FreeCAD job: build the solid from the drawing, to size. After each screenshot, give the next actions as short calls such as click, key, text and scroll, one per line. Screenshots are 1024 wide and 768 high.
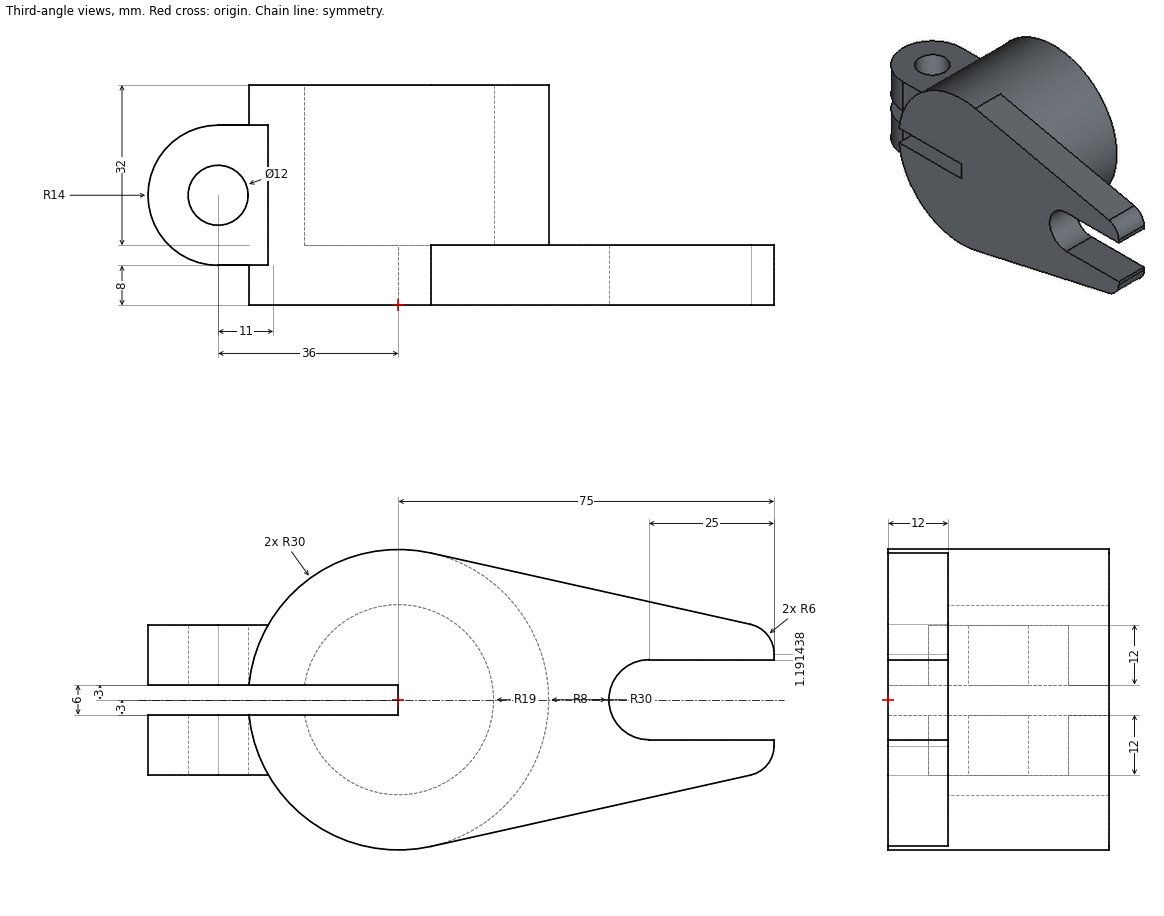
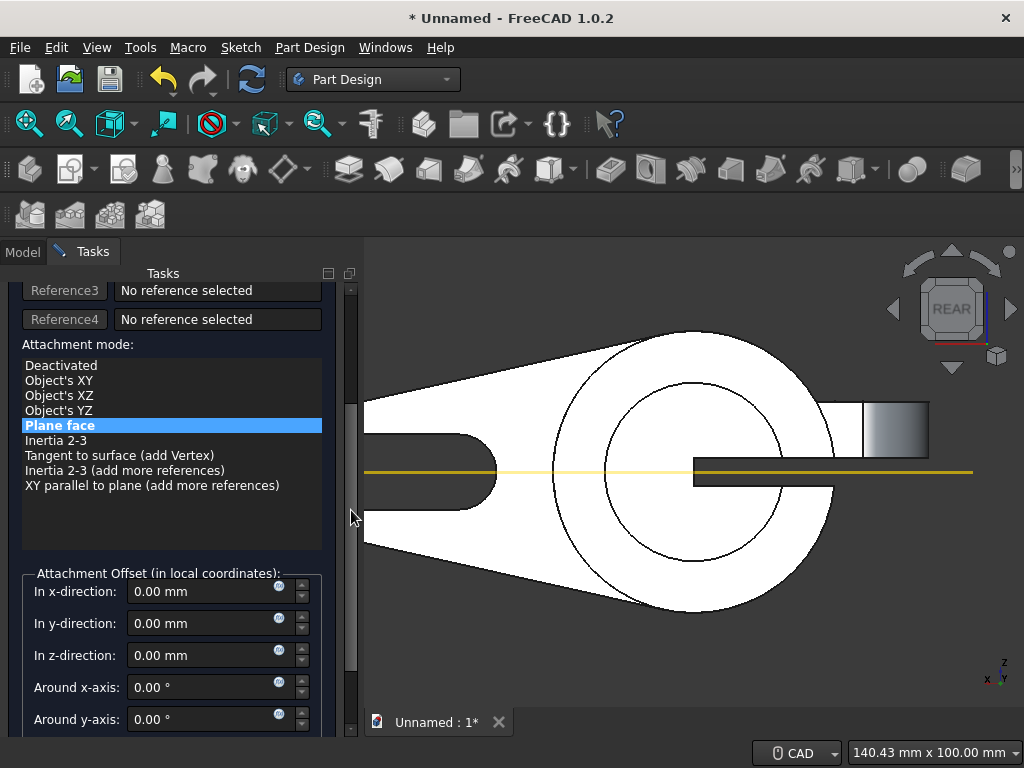
triple_click(210, 655)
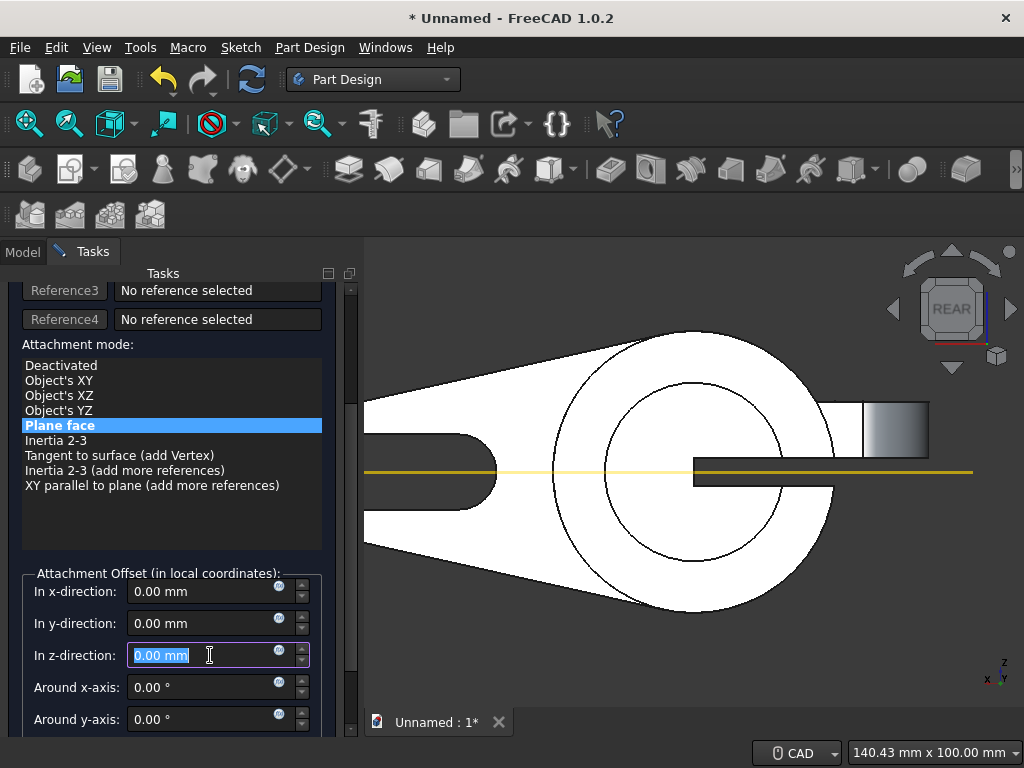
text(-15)
key(Tab)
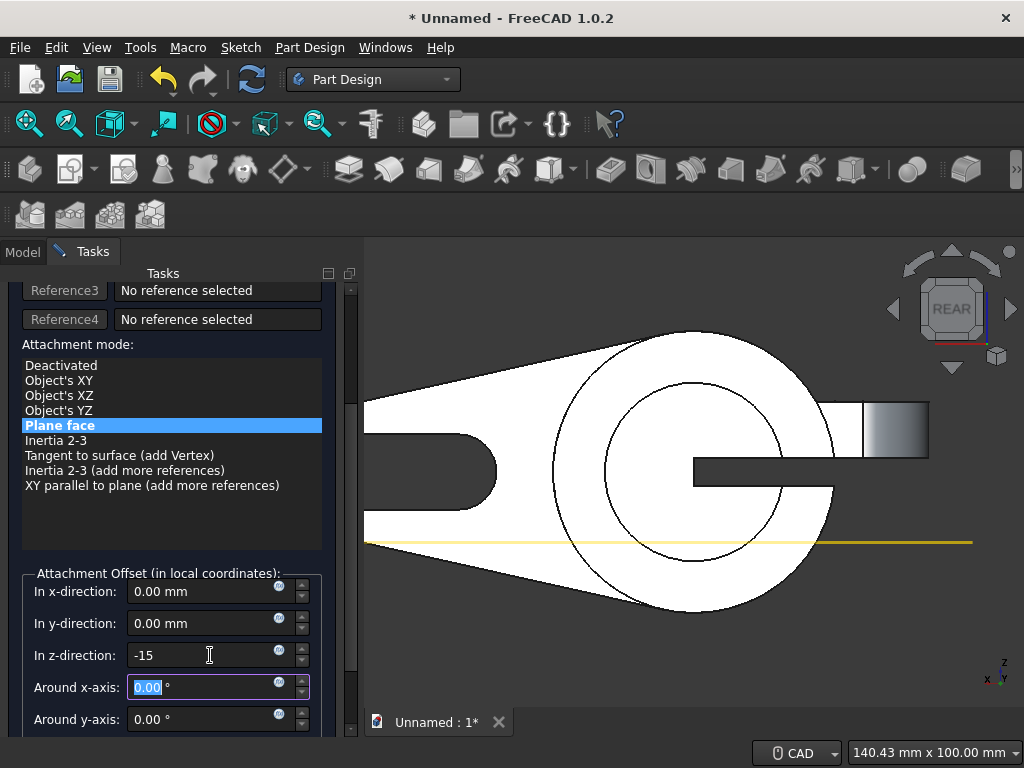
scroll(351, 510, up, 4)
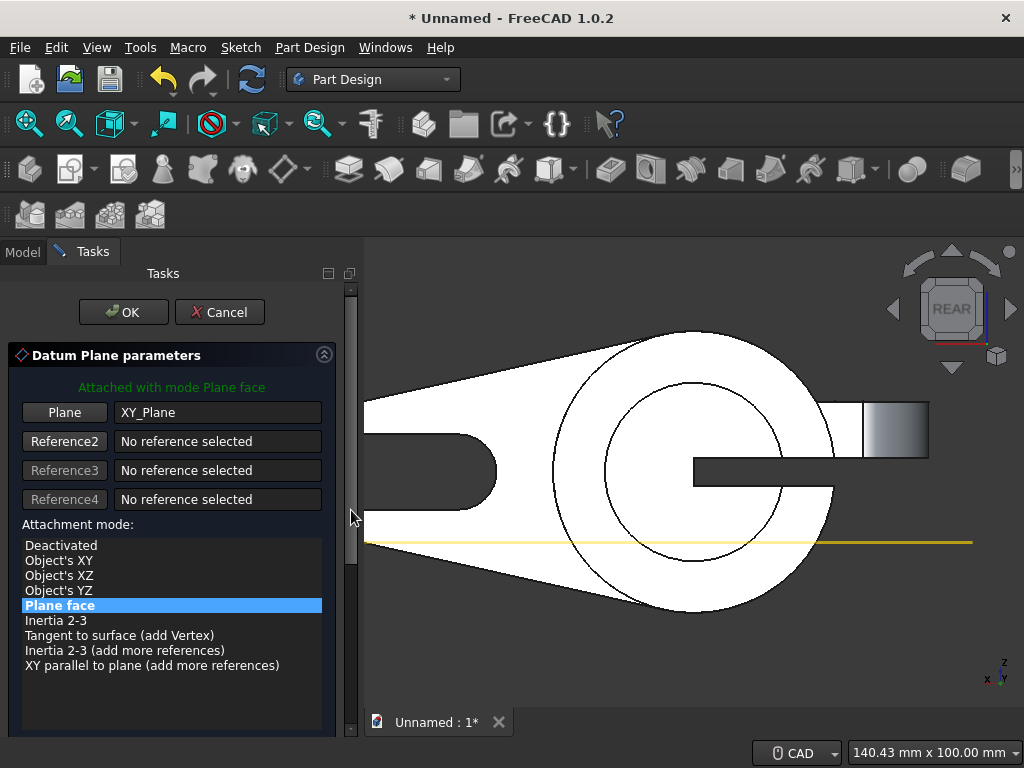
click(124, 312)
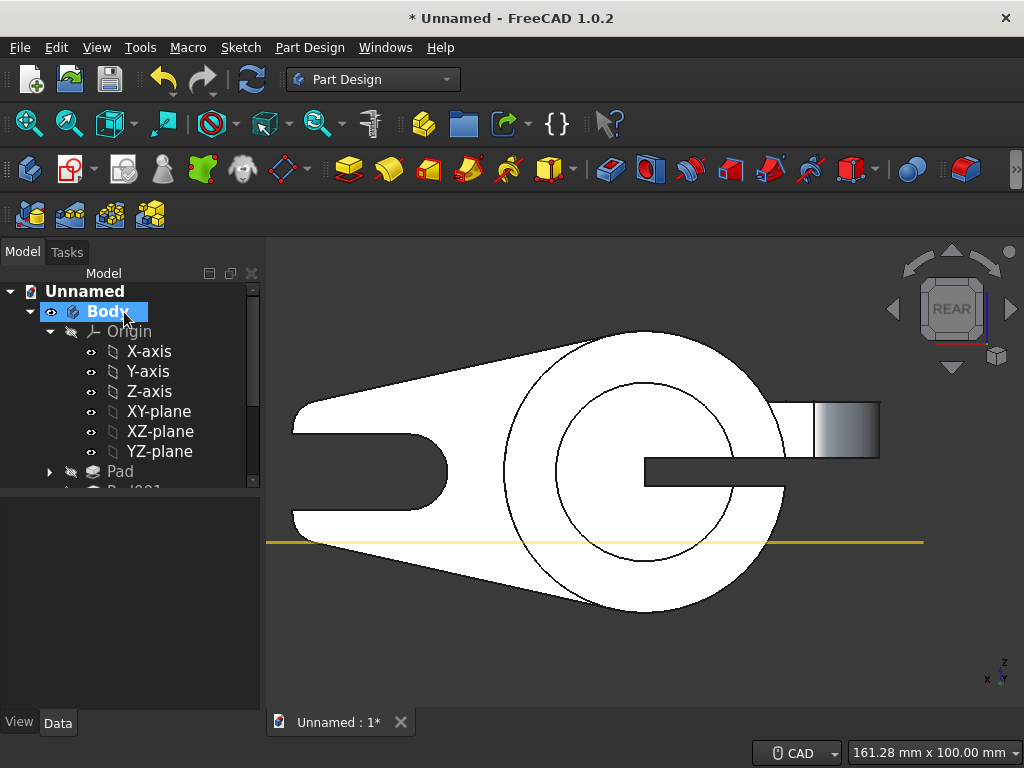
scroll(100, 387, down, 3)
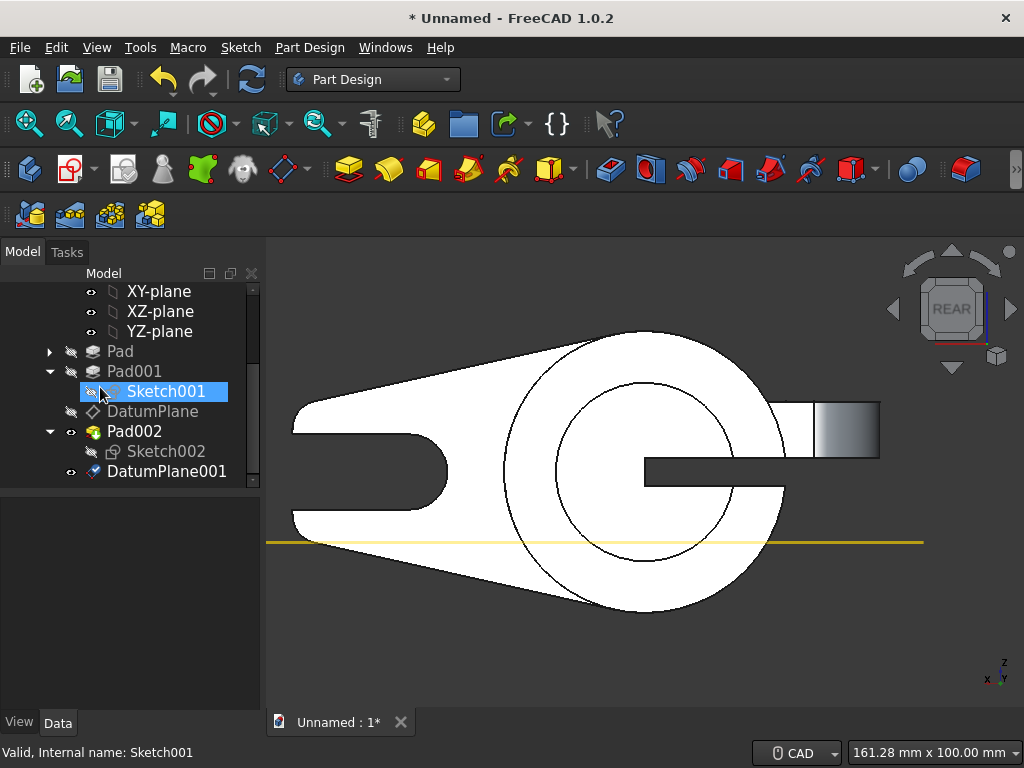
click(116, 472)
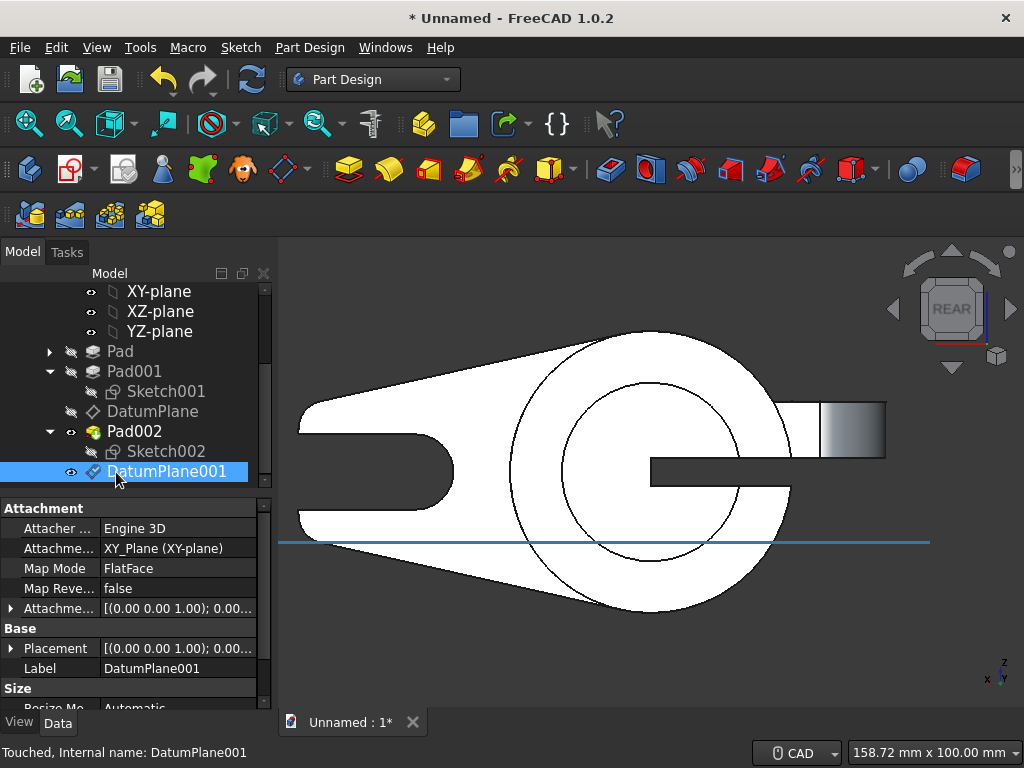
click(70, 170)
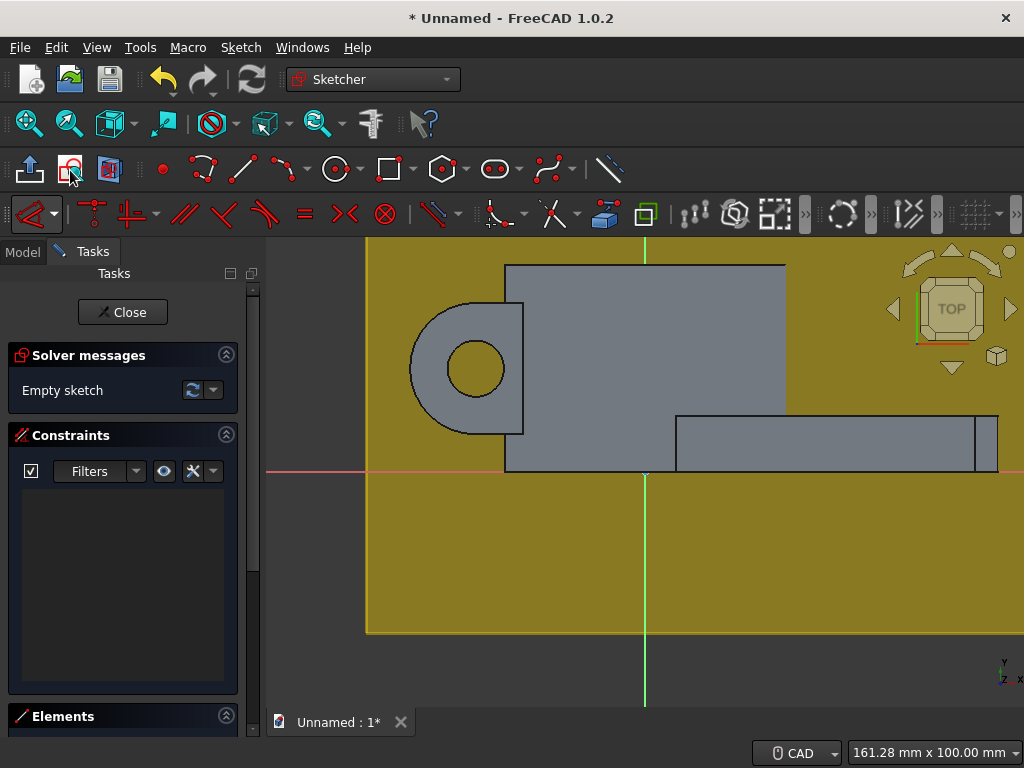
key(q)
key(s)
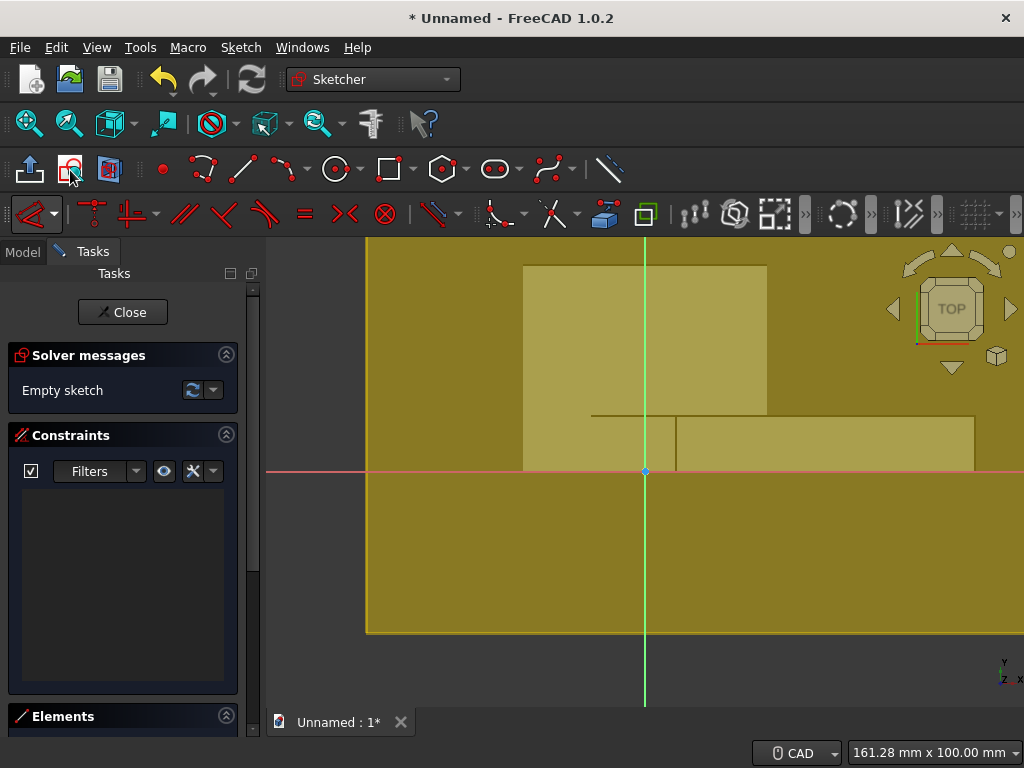
scroll(468, 284, up, 3)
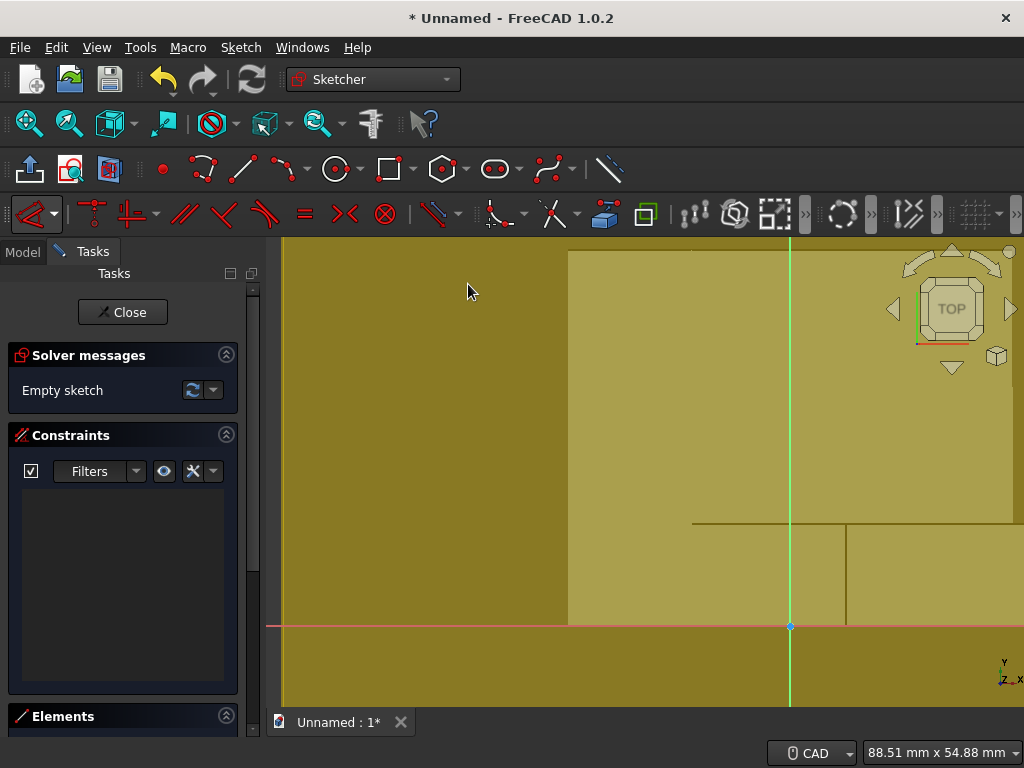
key(g)
key(m)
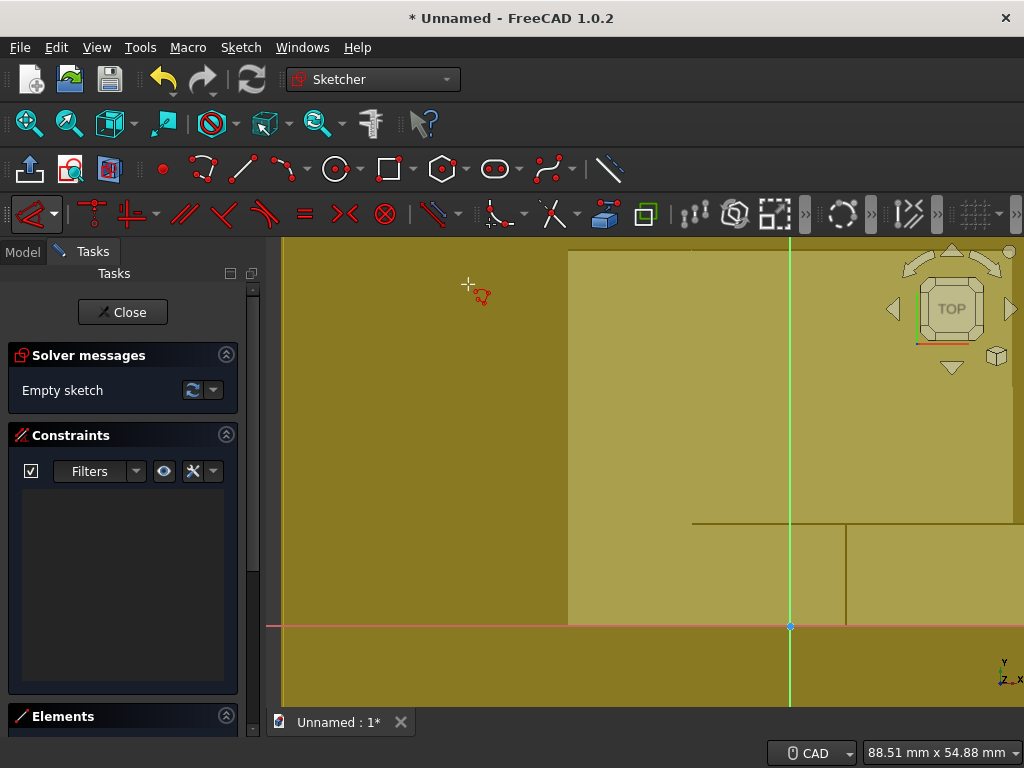
click(482, 558)
click(576, 558)
click(576, 318)
click(482, 318)
right_click(482, 318)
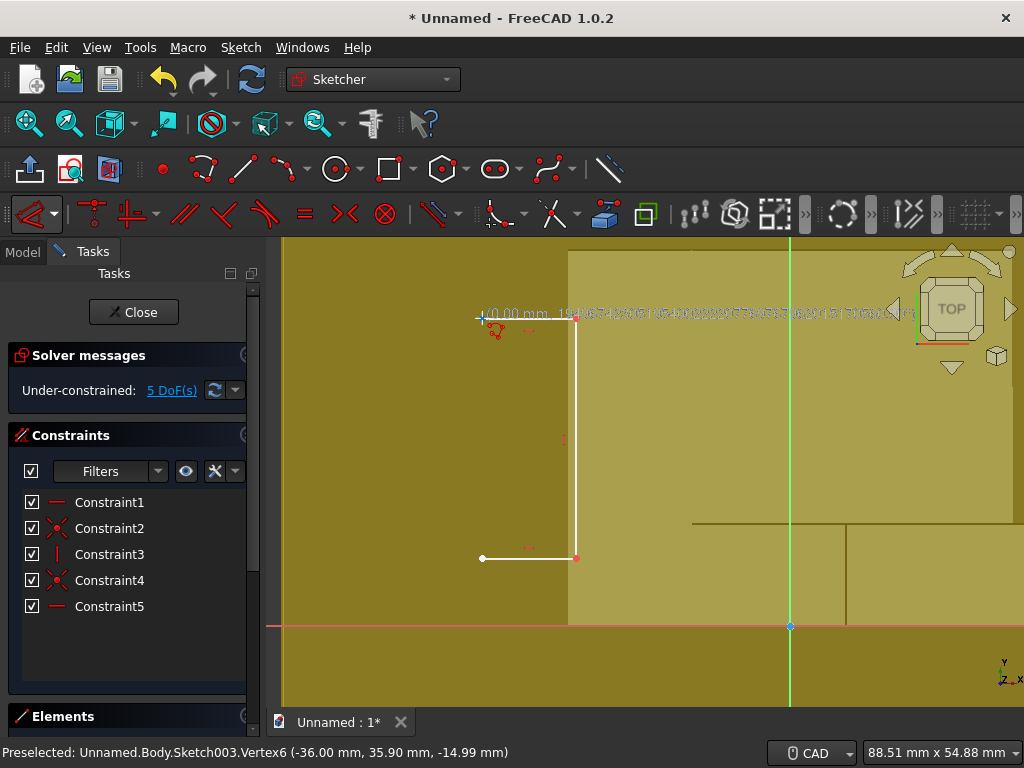
click(284, 170)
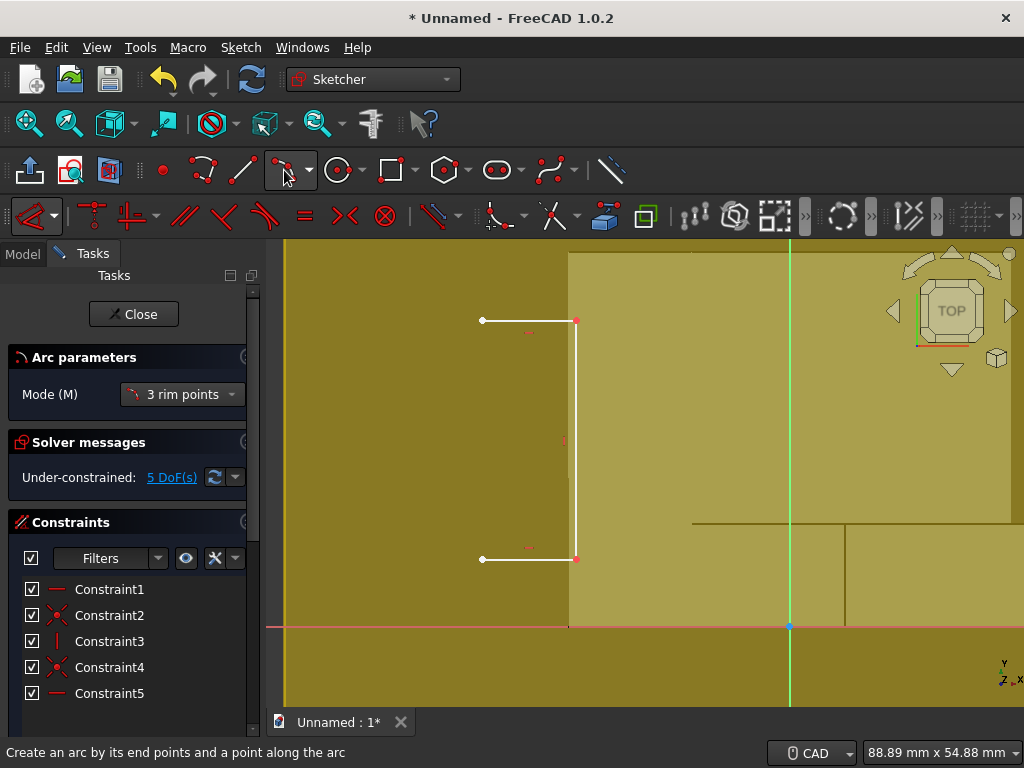
click(483, 321)
click(483, 560)
click(363, 439)